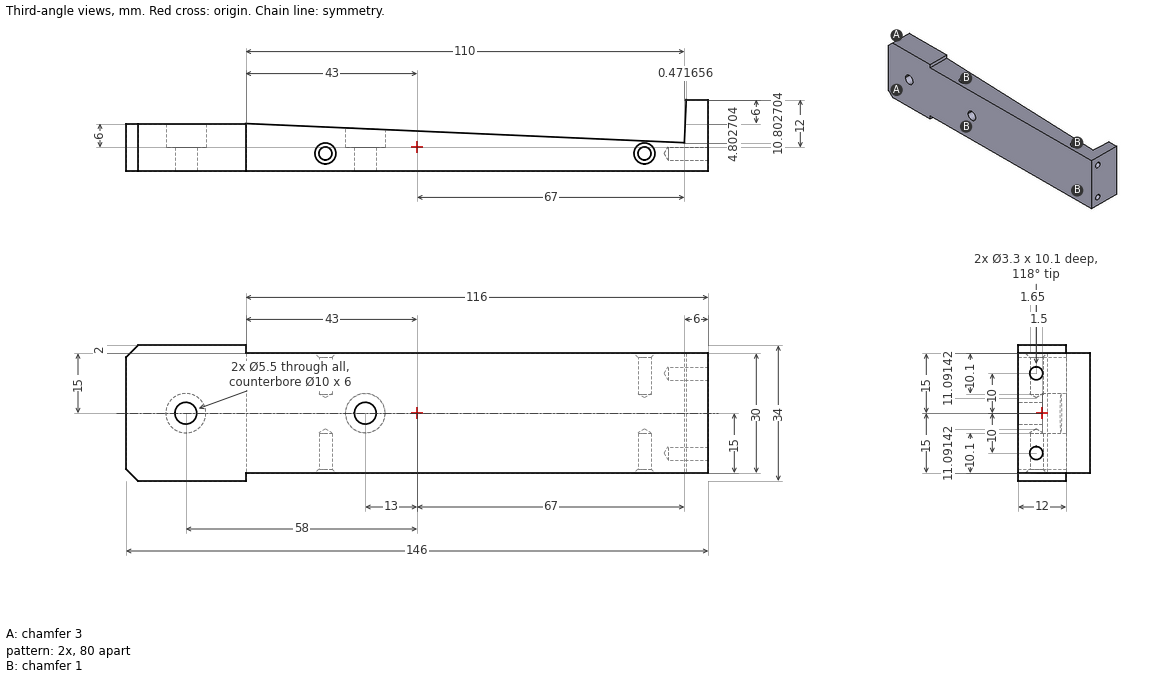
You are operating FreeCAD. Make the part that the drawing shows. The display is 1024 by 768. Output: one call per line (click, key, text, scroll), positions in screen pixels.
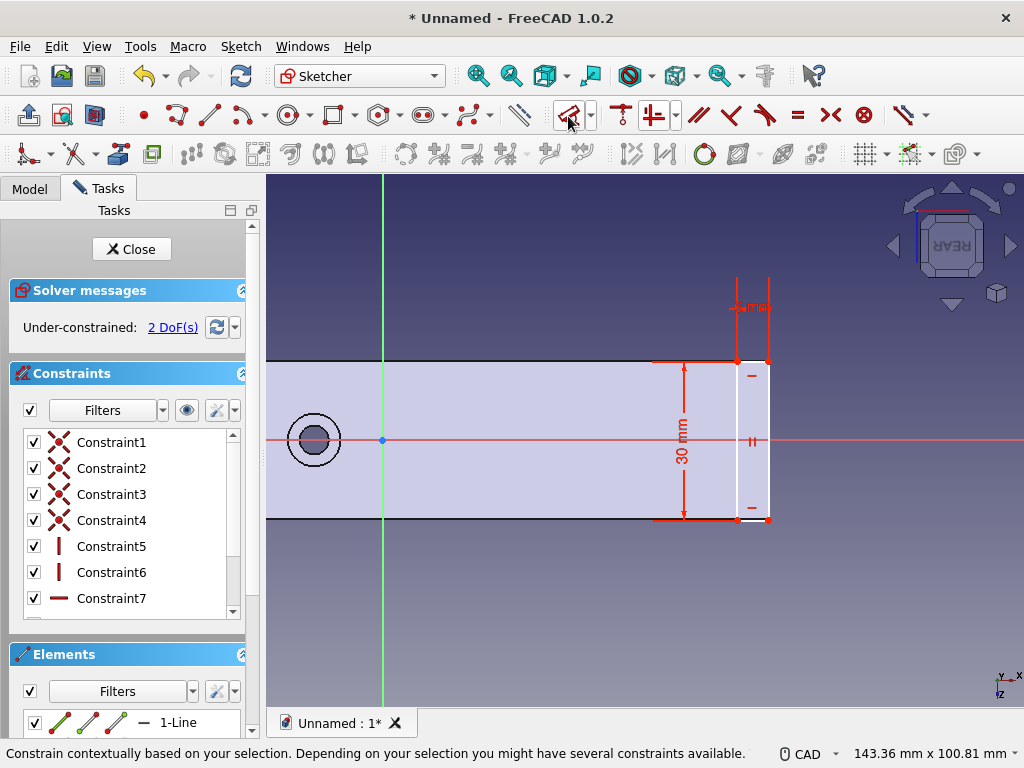
click(737, 362)
click(560, 328)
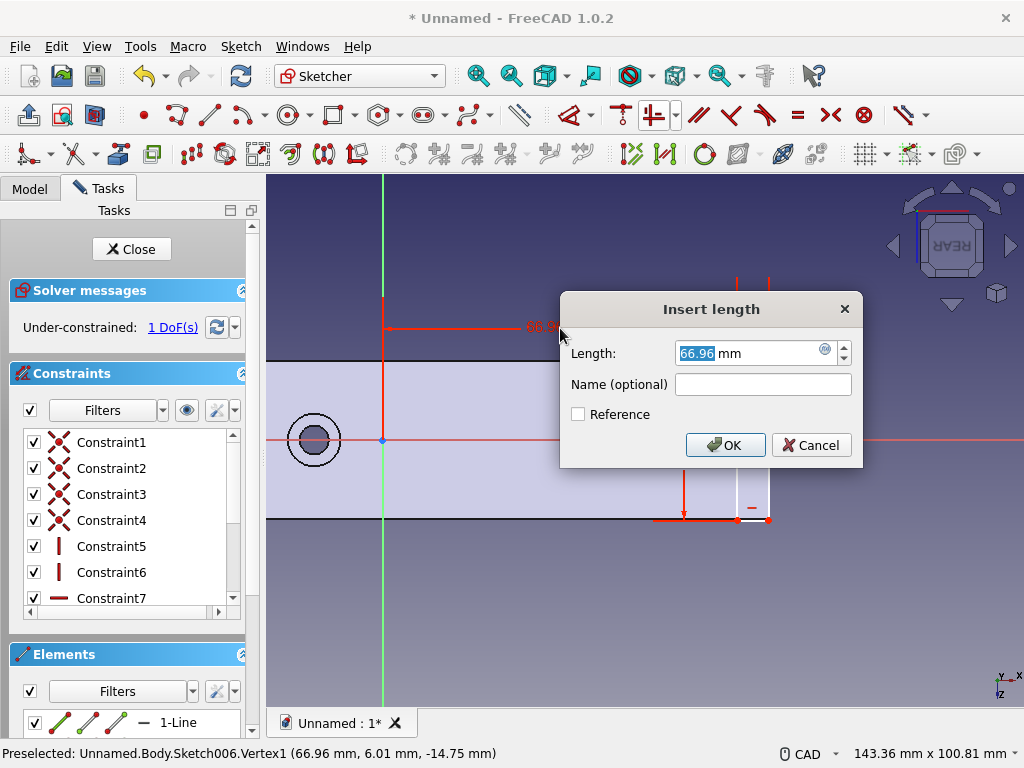
text(67)
key(Return)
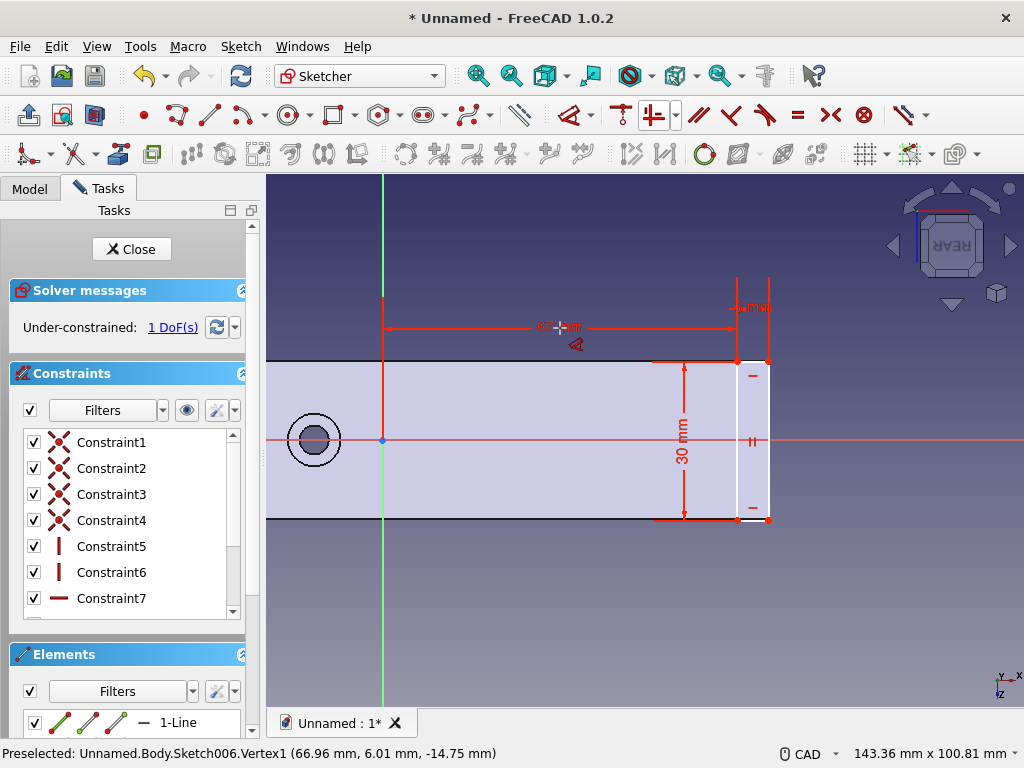
click(737, 362)
click(349, 401)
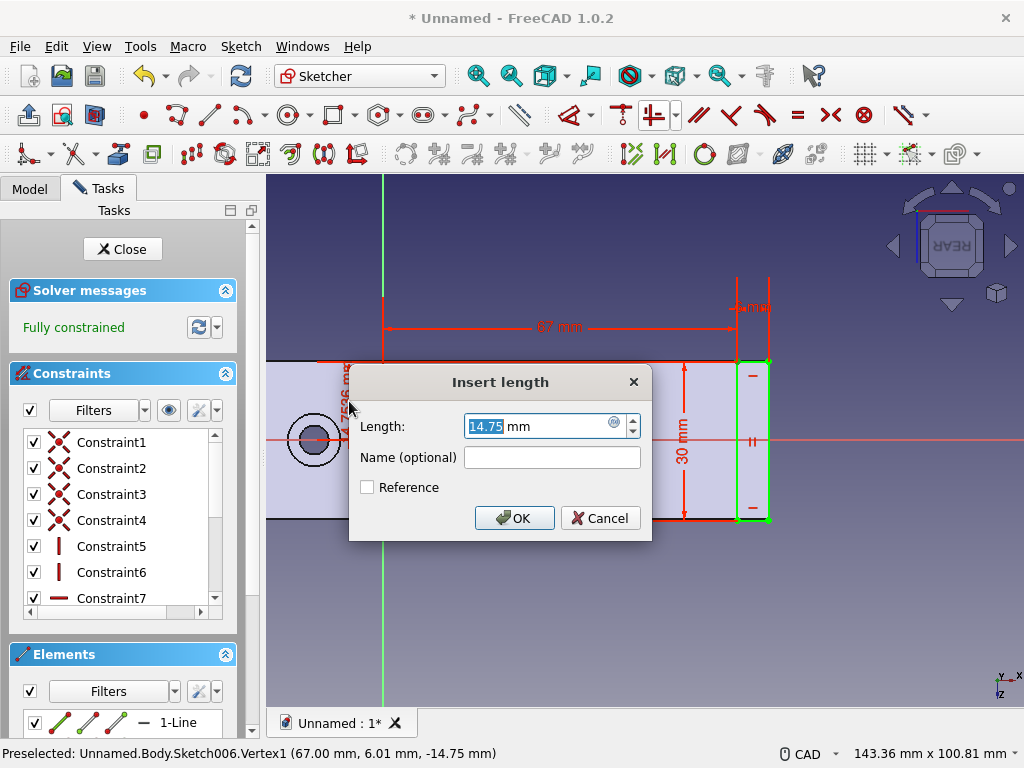
text(15)
key(Return)
key(Escape)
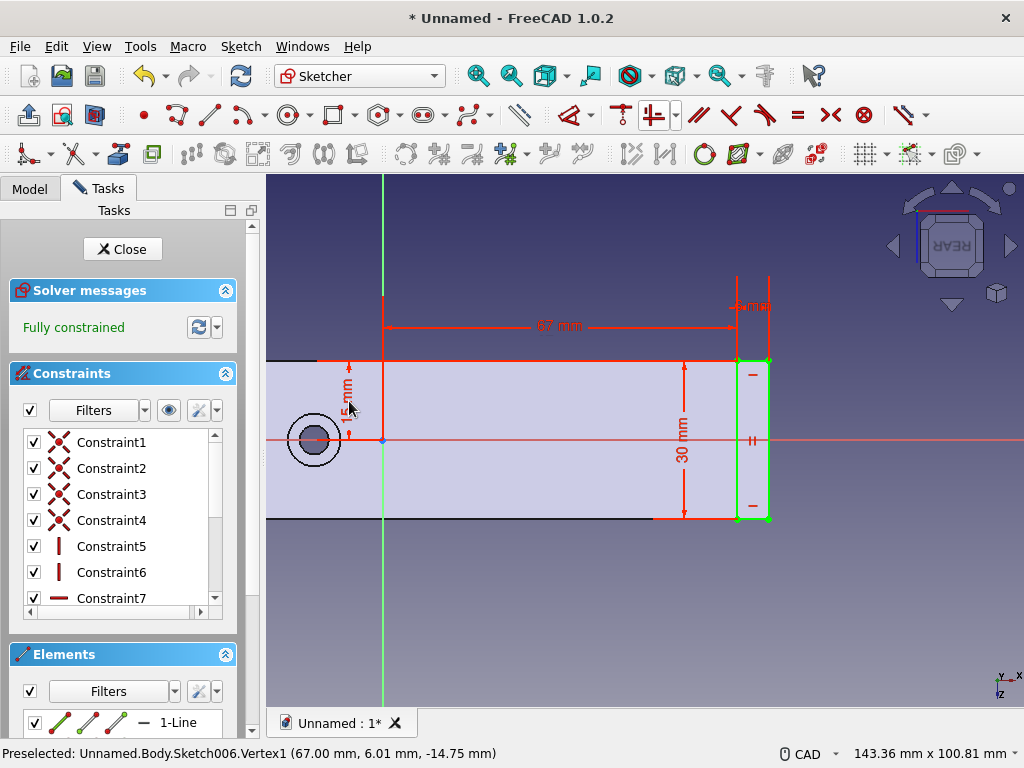
click(123, 249)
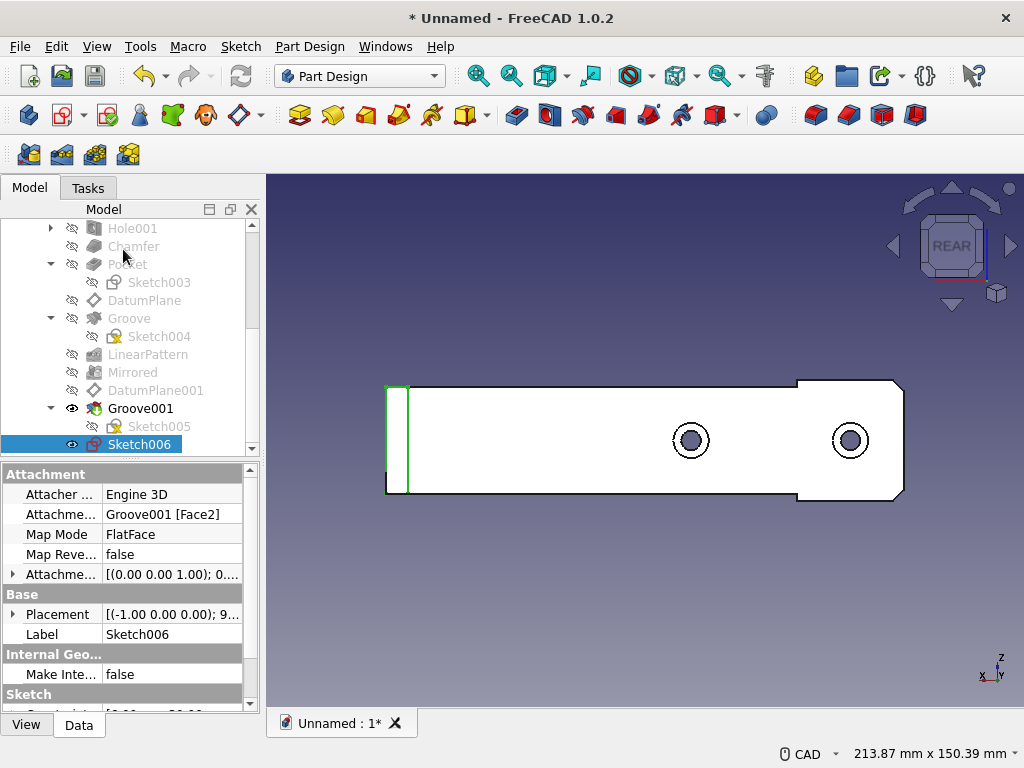
click(300, 116)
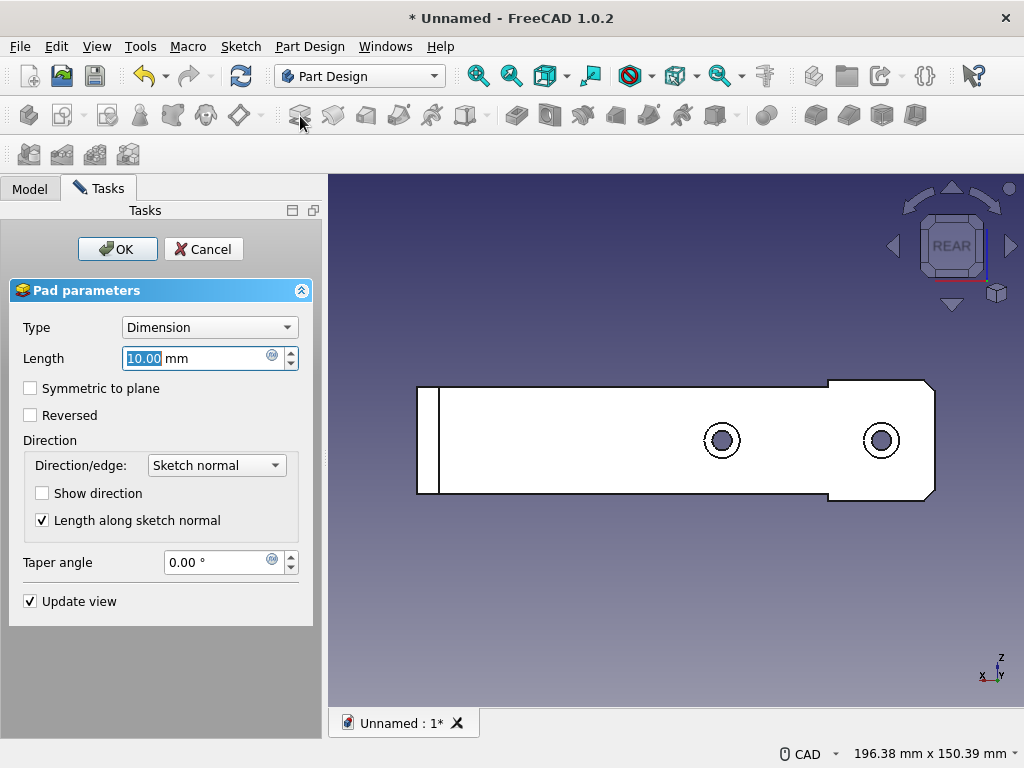
text(6)
key(Tab)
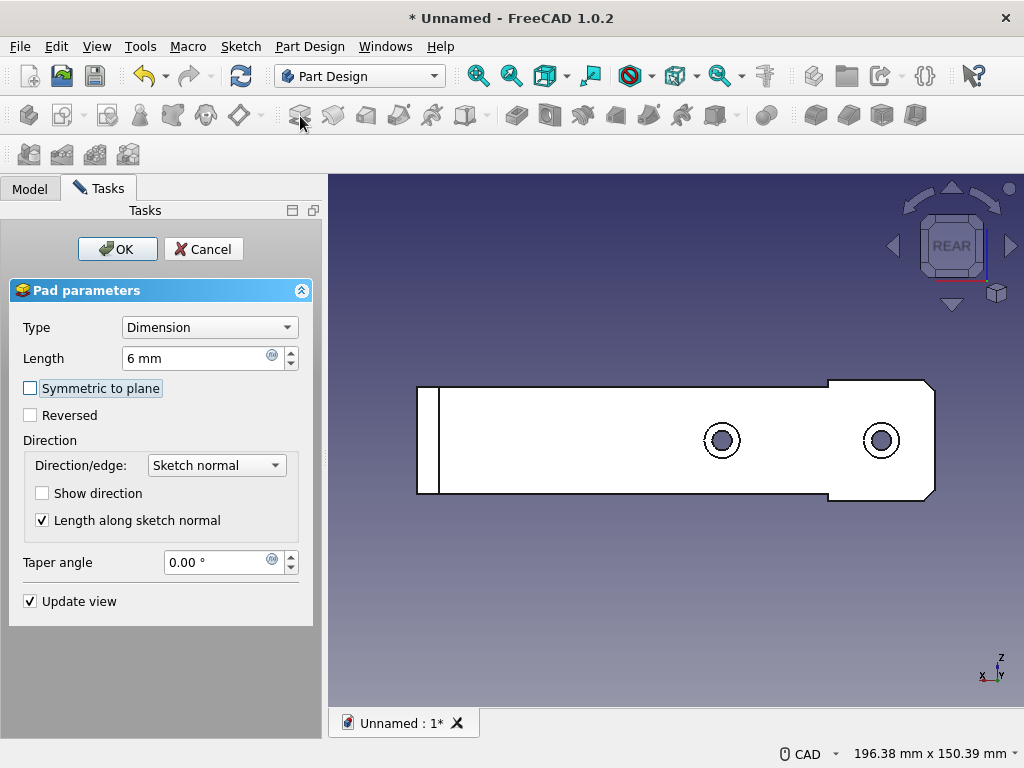
click(118, 249)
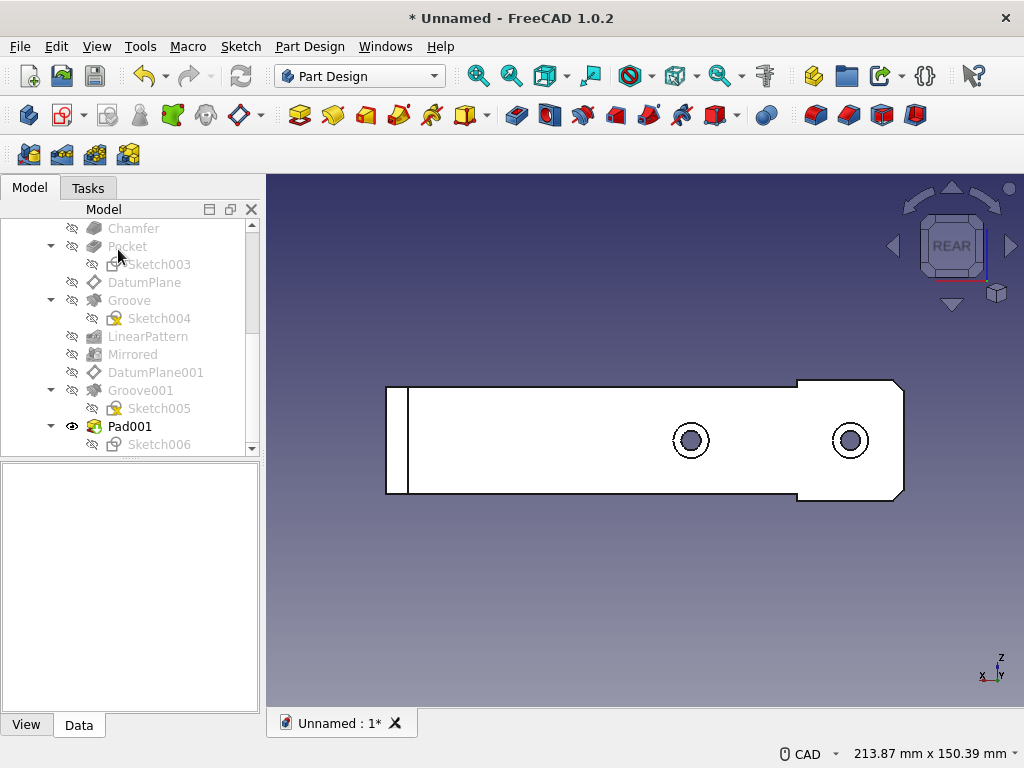
key(0)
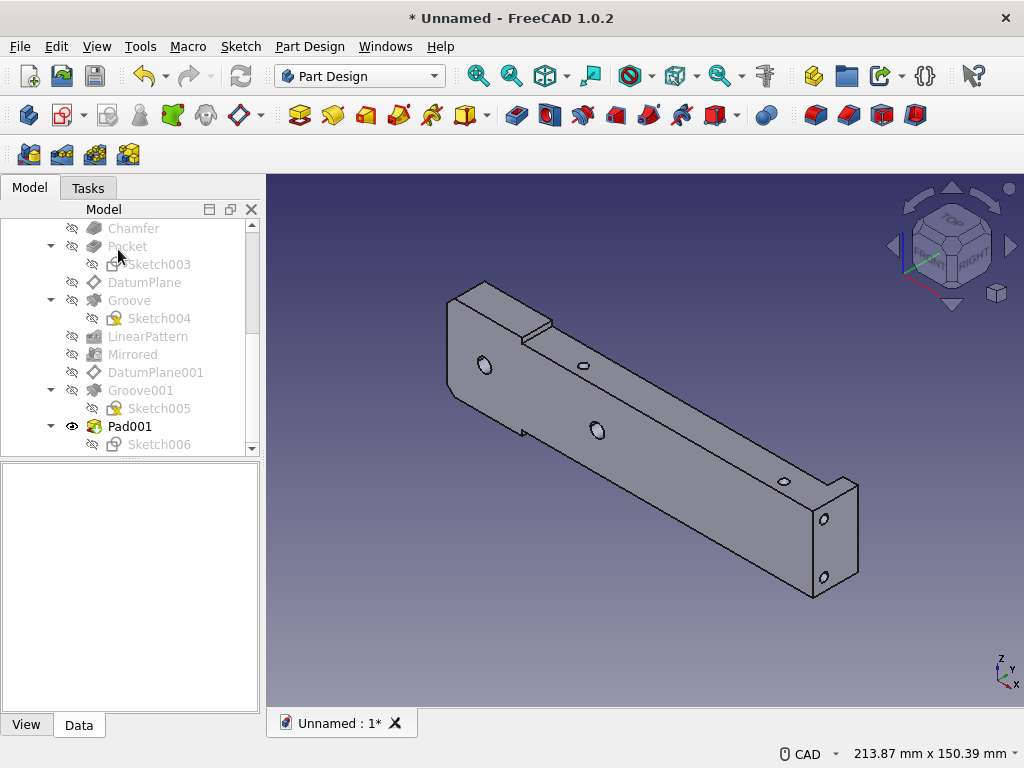
click(513, 314)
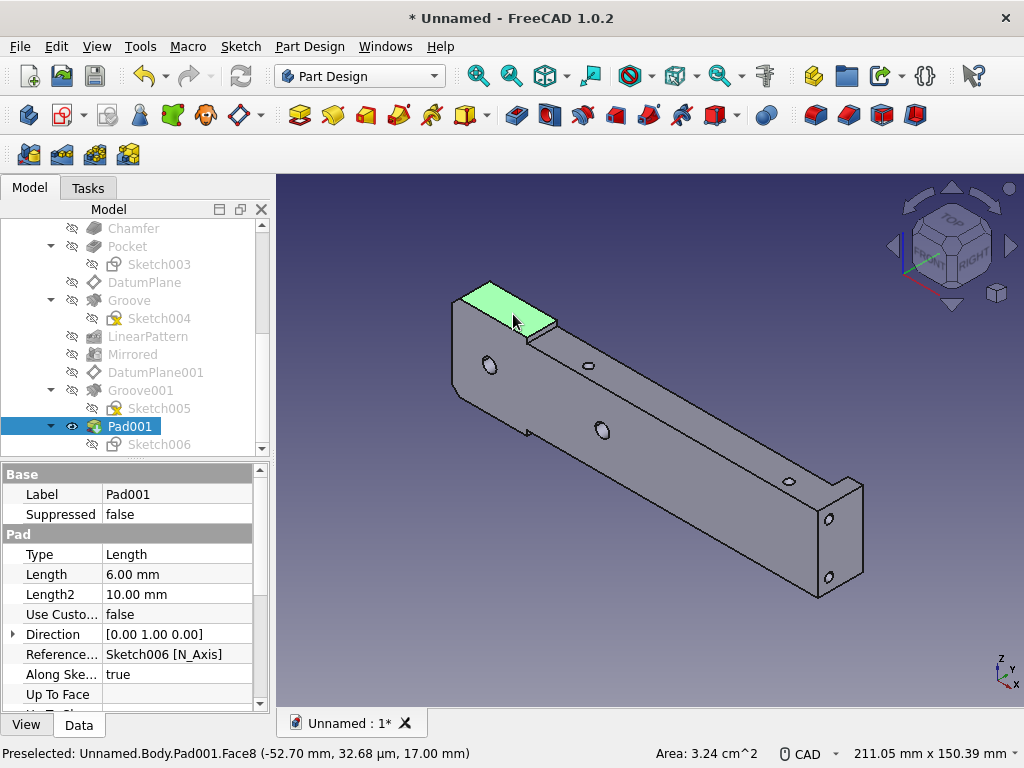
click(62, 116)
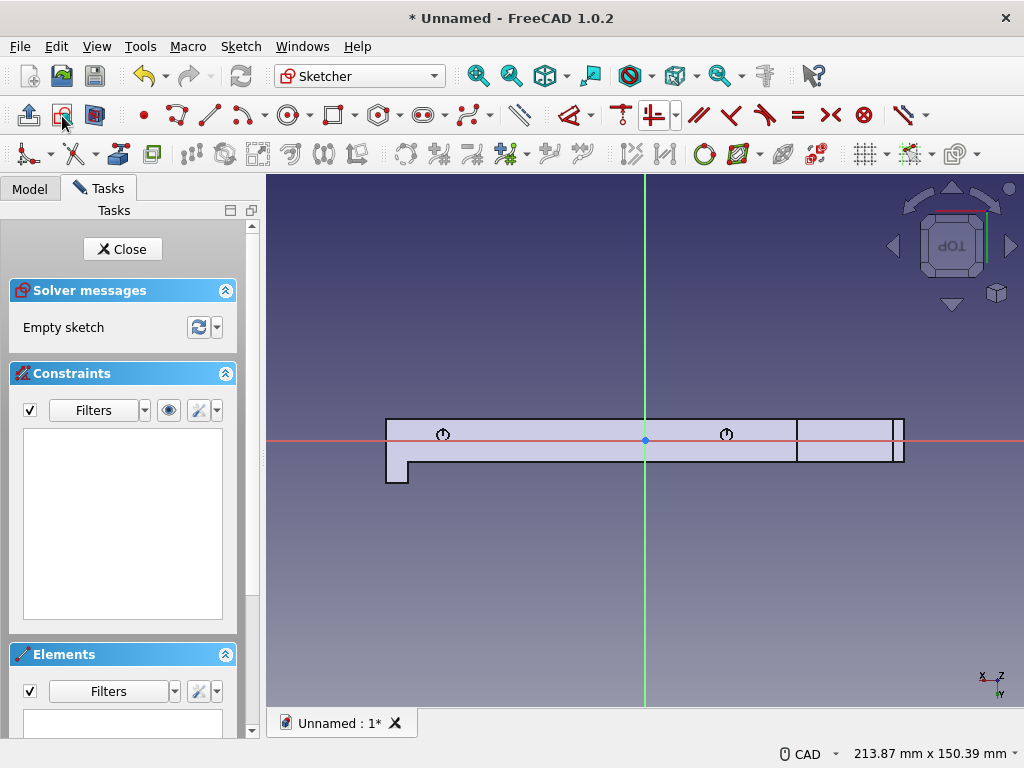
key(g)
key(m)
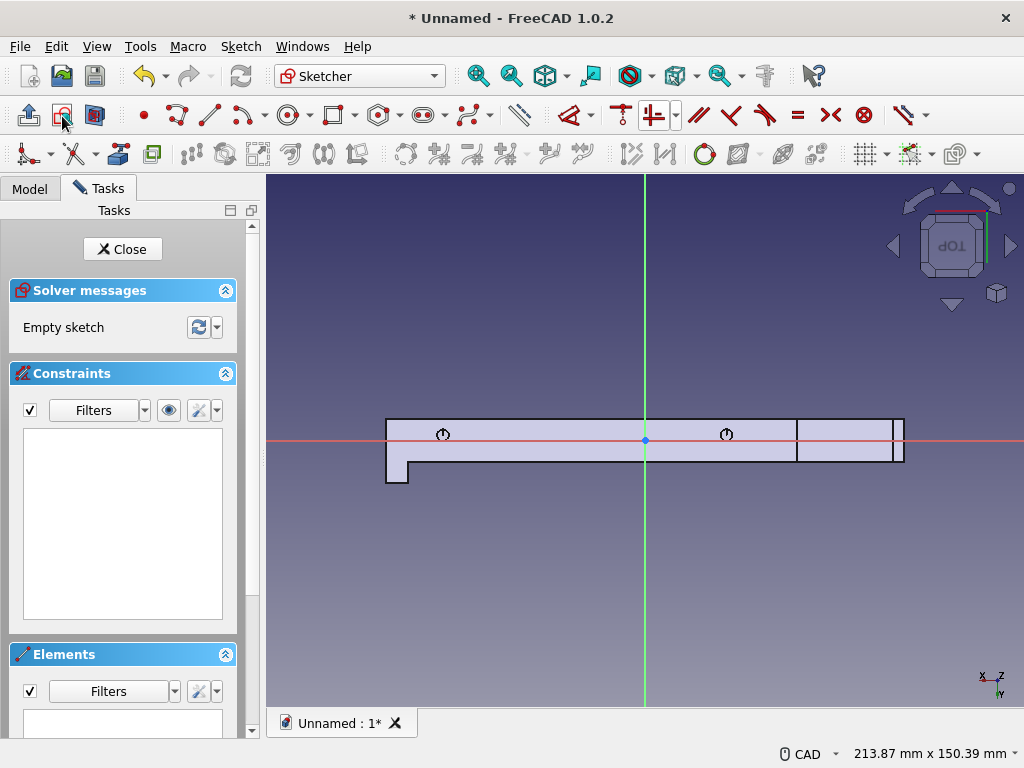
click(797, 462)